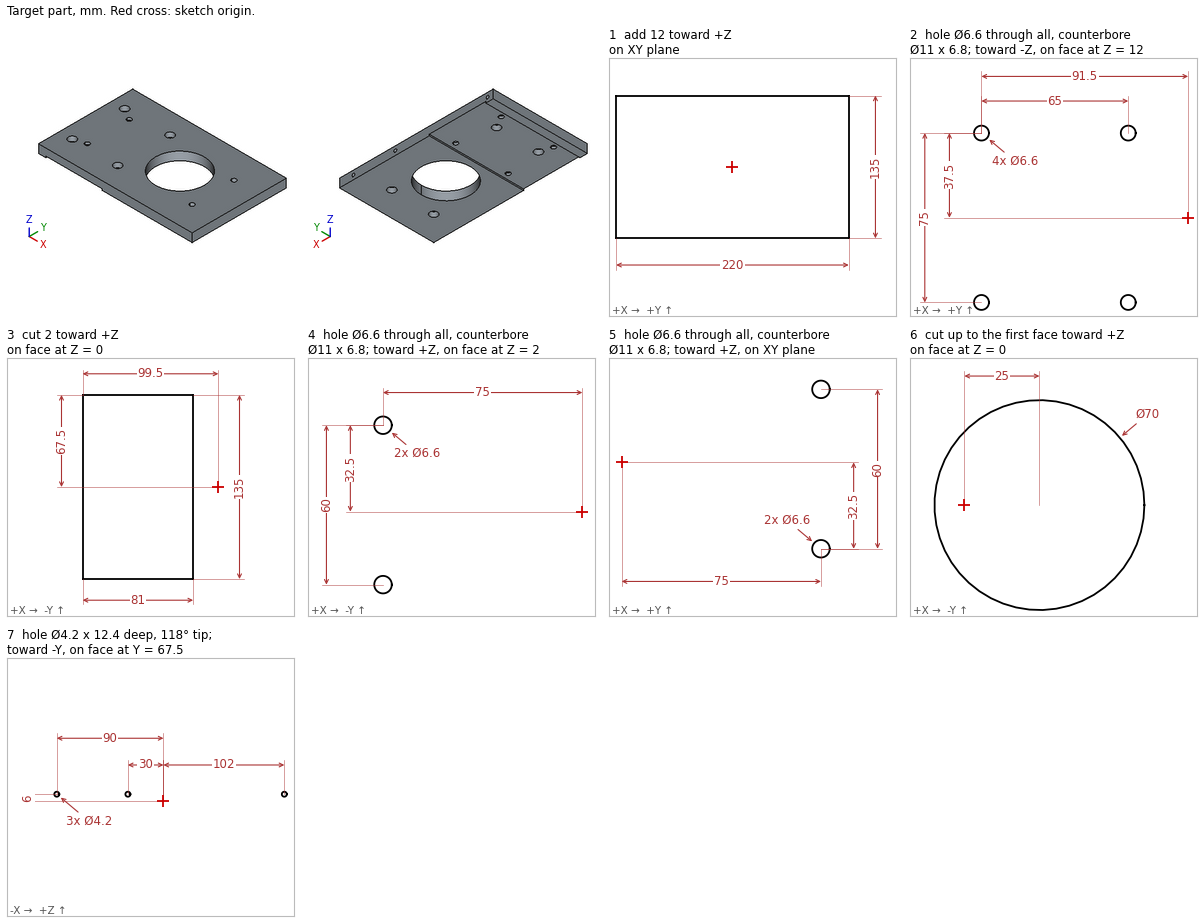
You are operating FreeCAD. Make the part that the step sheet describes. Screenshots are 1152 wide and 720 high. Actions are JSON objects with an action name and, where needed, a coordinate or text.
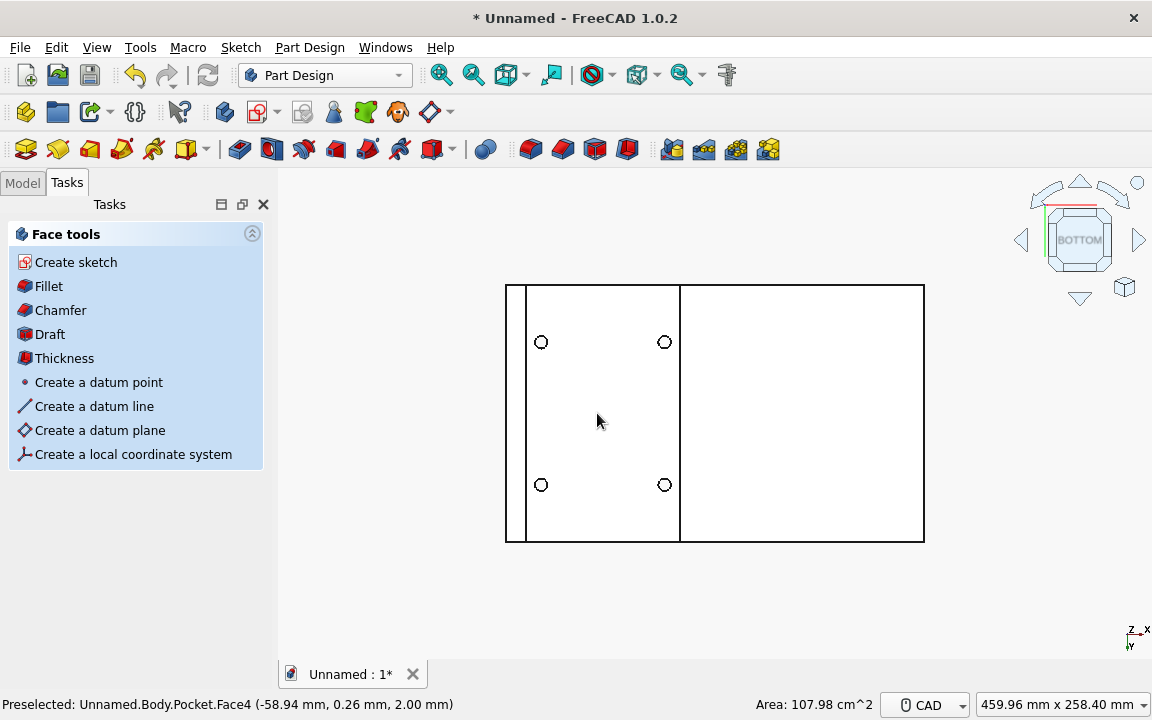
{"action": "left_click", "coordinate": [258, 112]}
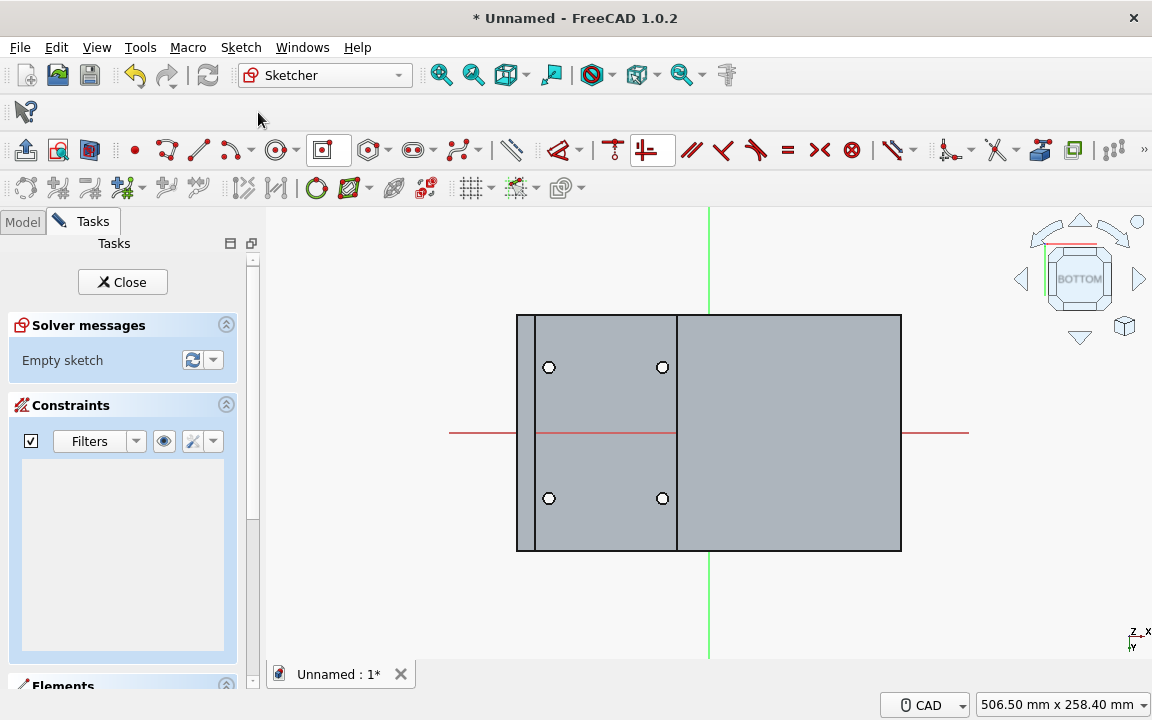
{"action": "key", "text": "q s"}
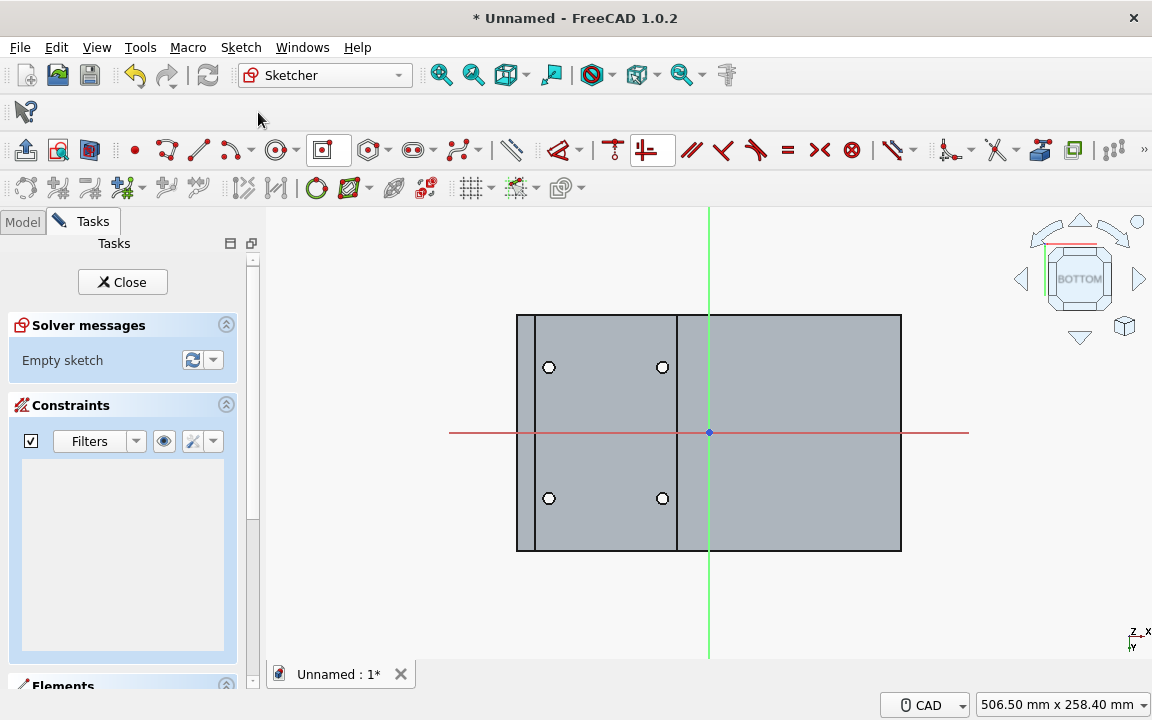
{"action": "scroll", "coordinate": [641, 425], "scroll_direction": "up", "scroll_amount": 4}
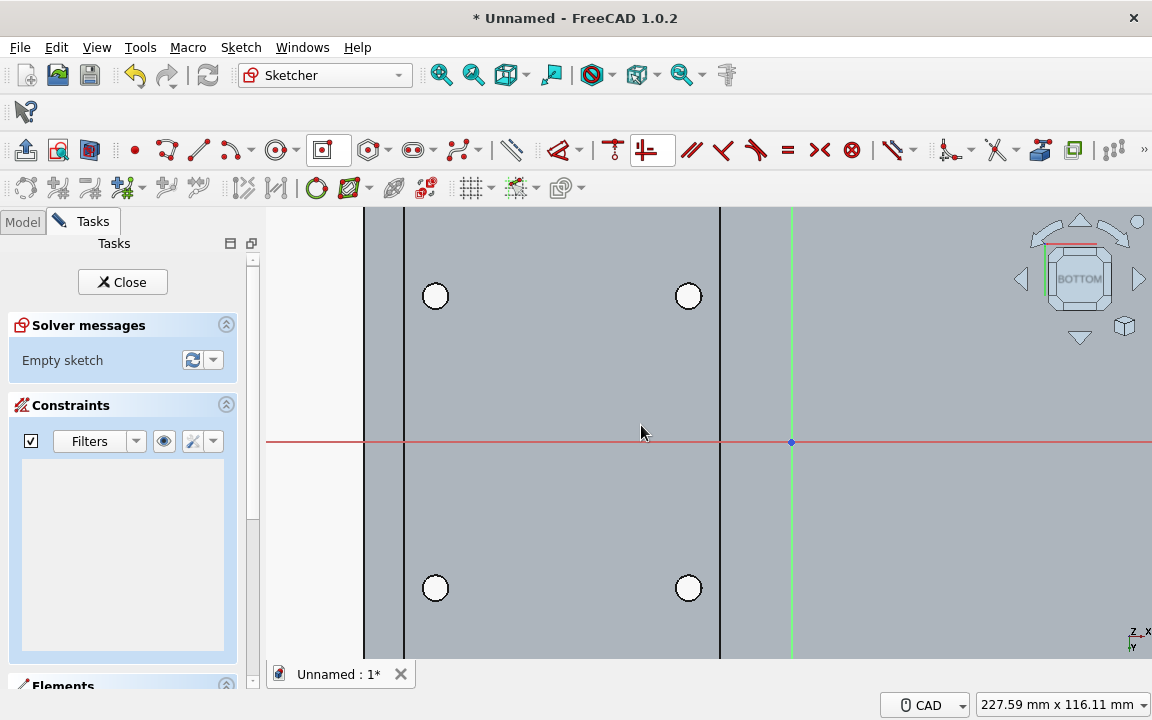
{"action": "left_click", "coordinate": [276, 150]}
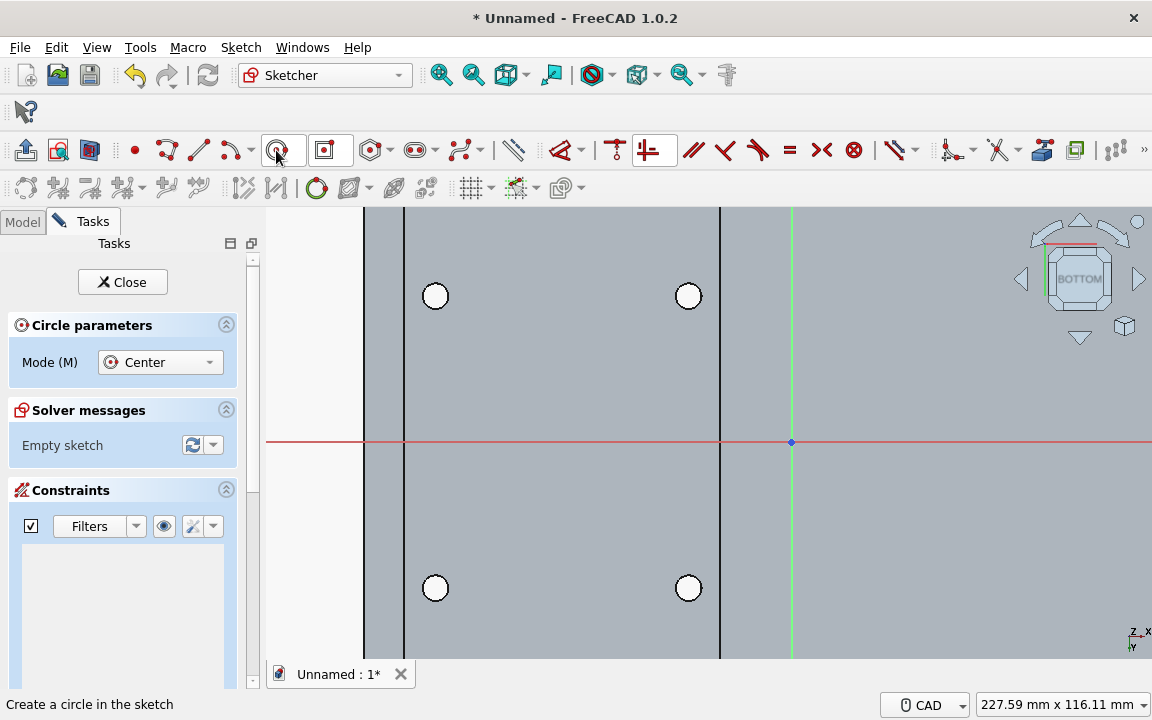
{"action": "scroll", "coordinate": [500, 316], "scroll_direction": "up", "scroll_amount": 3}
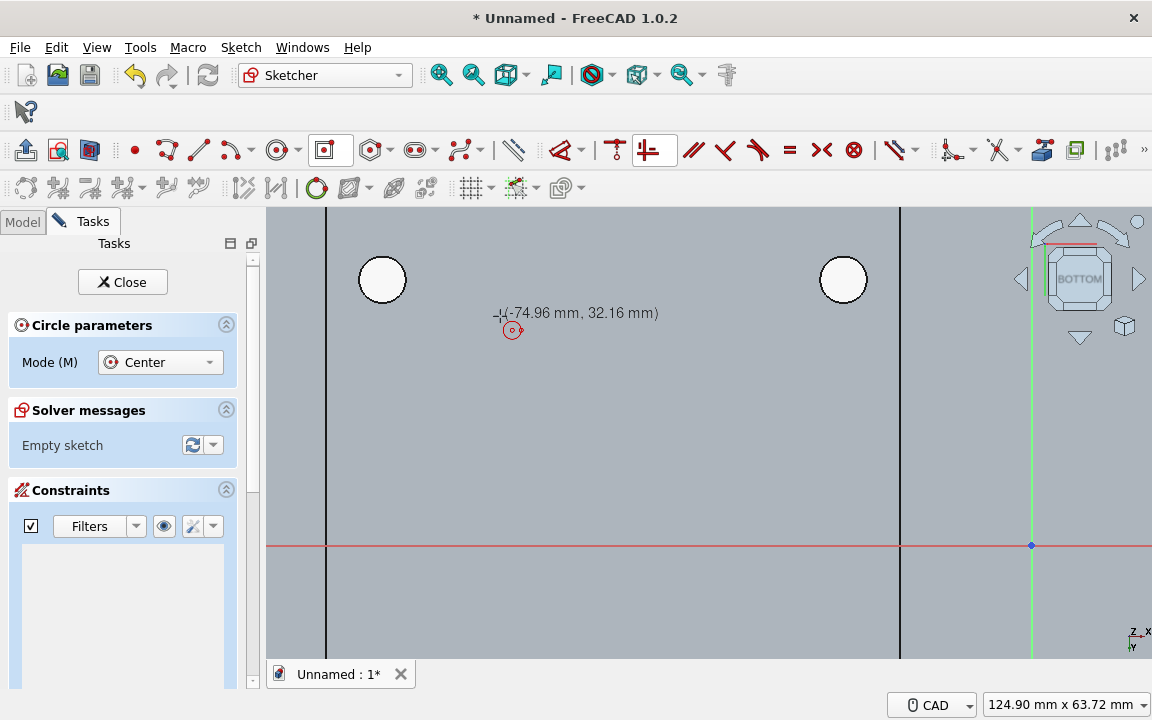
{"action": "left_click", "coordinate": [499, 315]}
{"action": "mouse_move", "coordinate": [516, 299]}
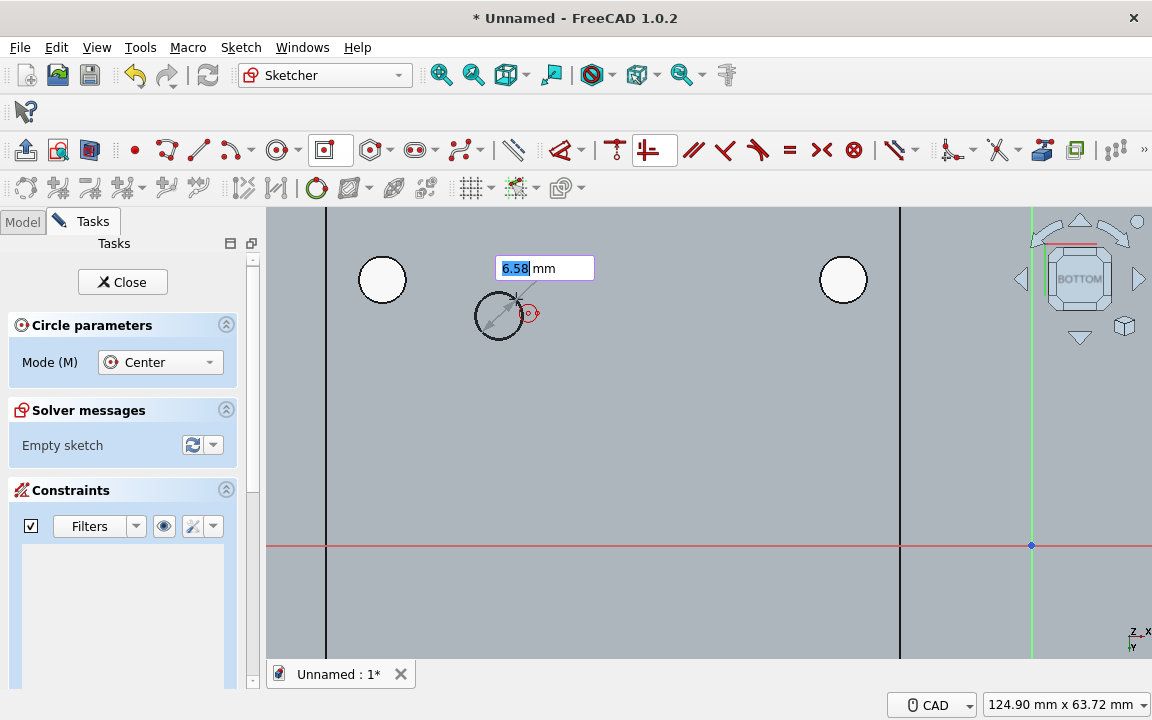
{"action": "type", "text": "6.6"}
{"action": "key", "text": "Return"}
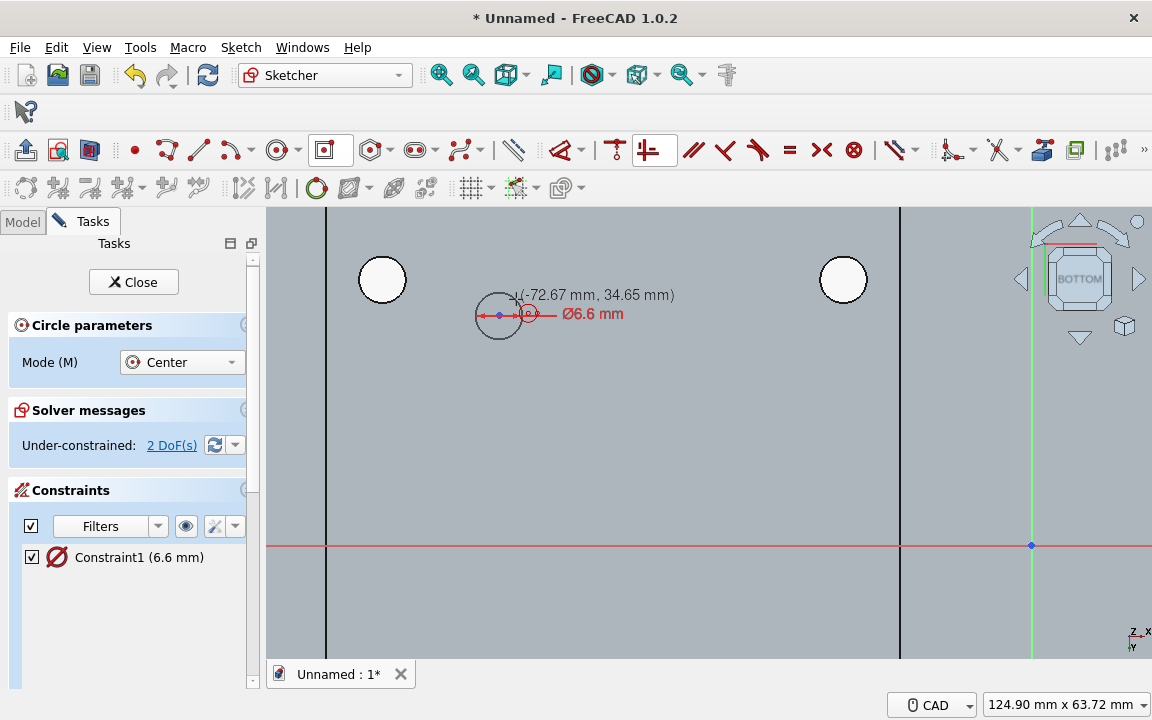
{"action": "scroll", "coordinate": [503, 317], "scroll_direction": "down", "scroll_amount": 3}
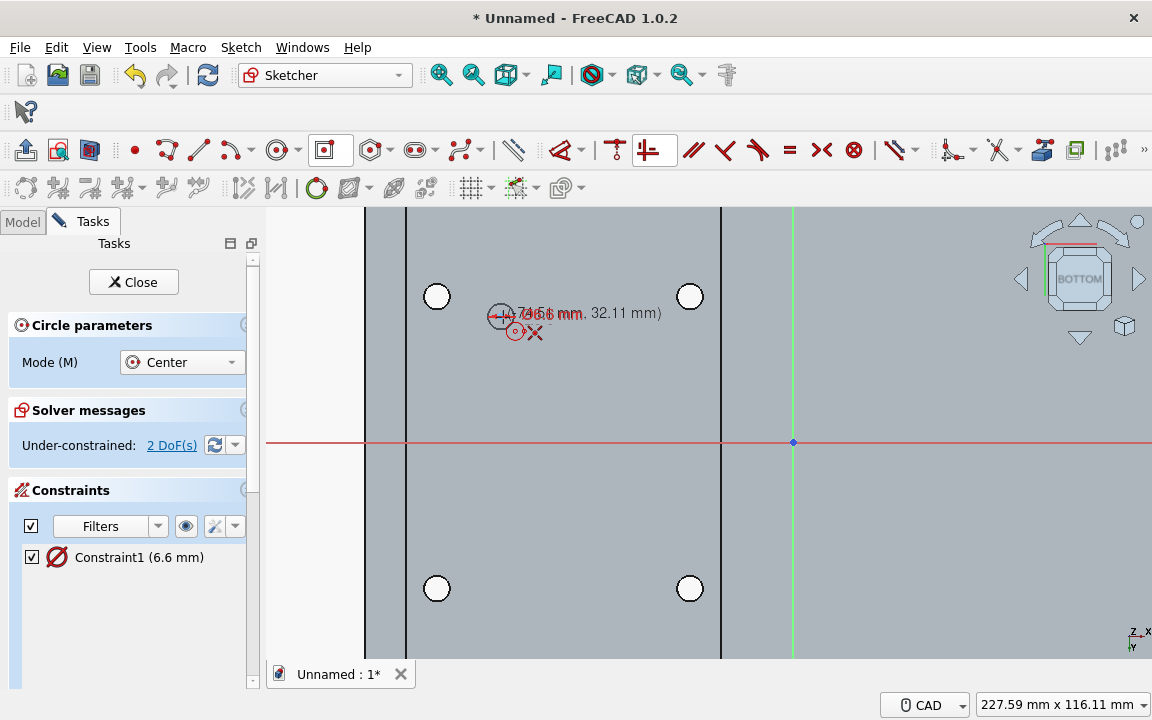
{"action": "scroll", "coordinate": [501, 550], "scroll_direction": "up", "scroll_amount": 3}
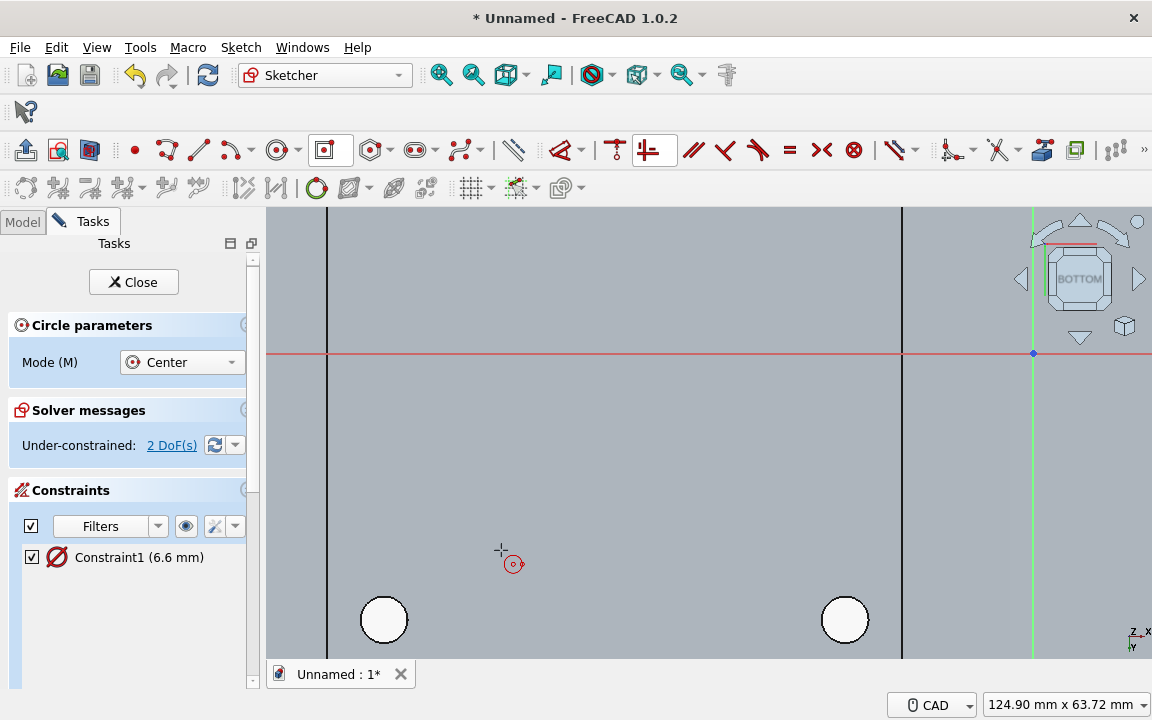
{"action": "left_click", "coordinate": [501, 549]}
{"action": "mouse_move", "coordinate": [518, 532]}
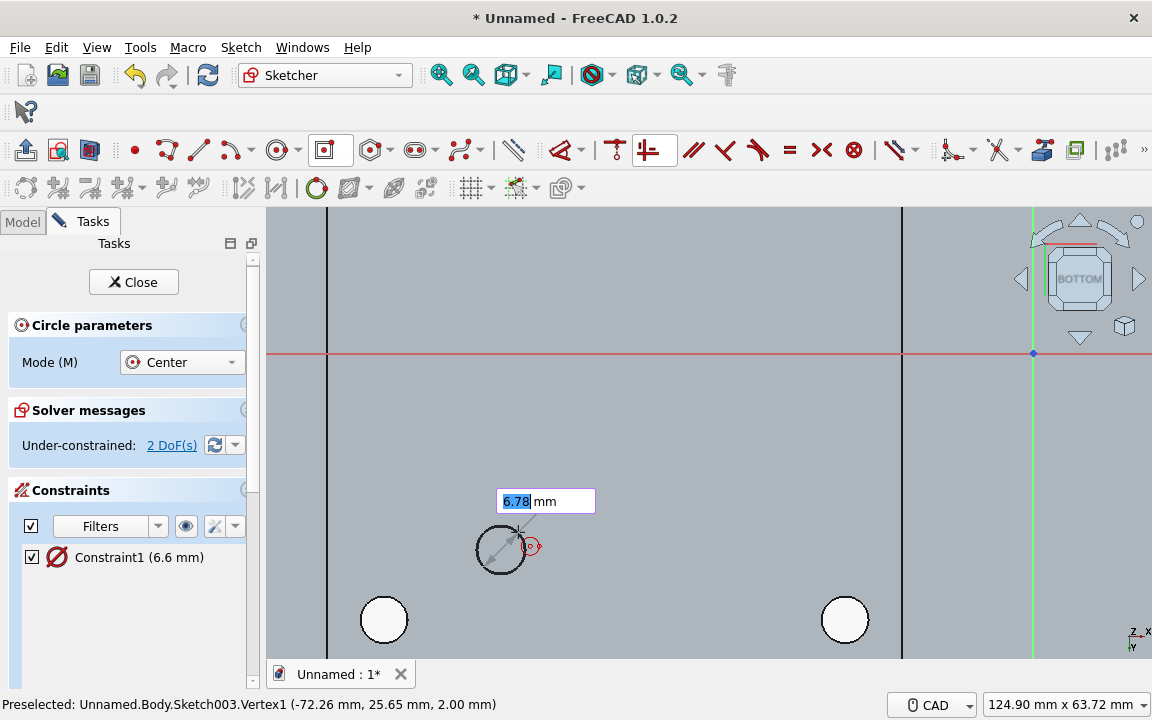
{"action": "type", "text": "6.6"}
{"action": "key", "text": "Return"}
{"action": "key", "text": "Escape"}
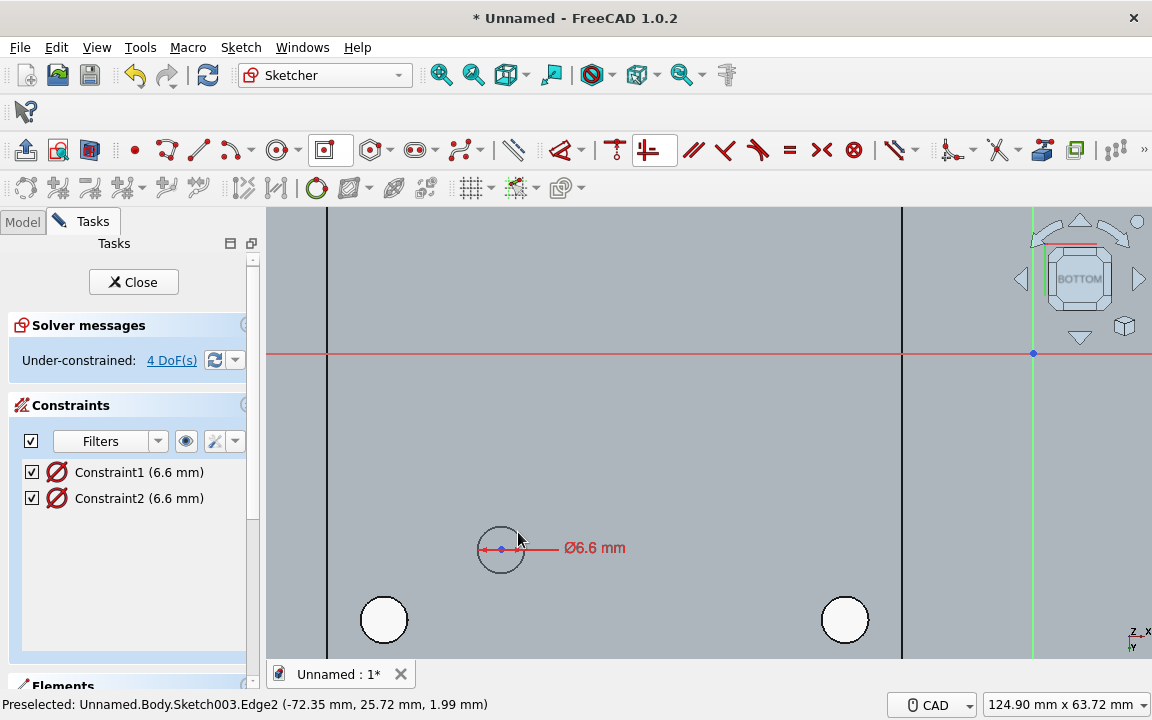
{"action": "scroll", "coordinate": [501, 551], "scroll_direction": "down", "scroll_amount": 3}